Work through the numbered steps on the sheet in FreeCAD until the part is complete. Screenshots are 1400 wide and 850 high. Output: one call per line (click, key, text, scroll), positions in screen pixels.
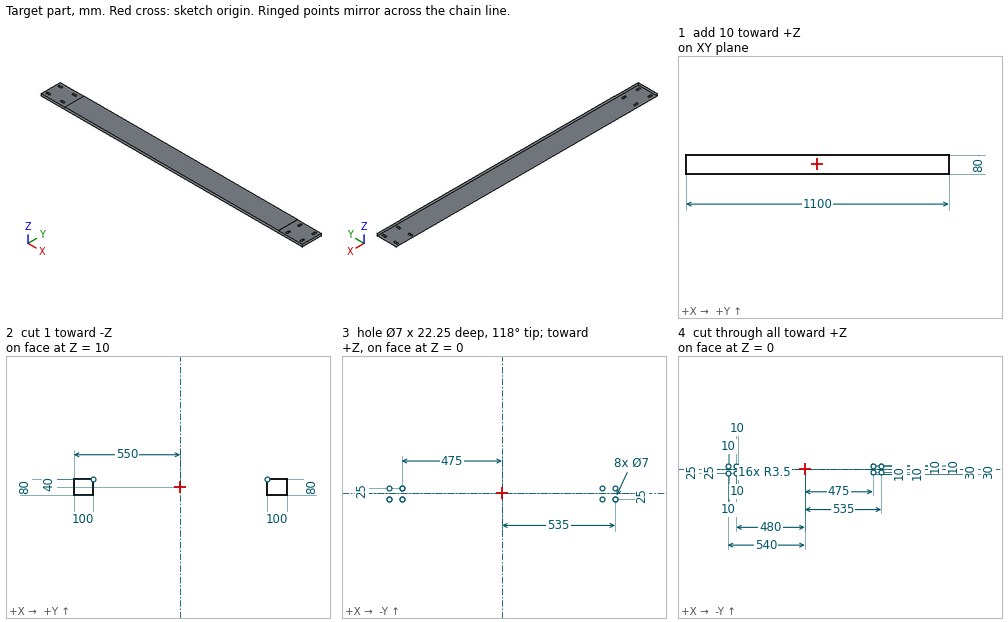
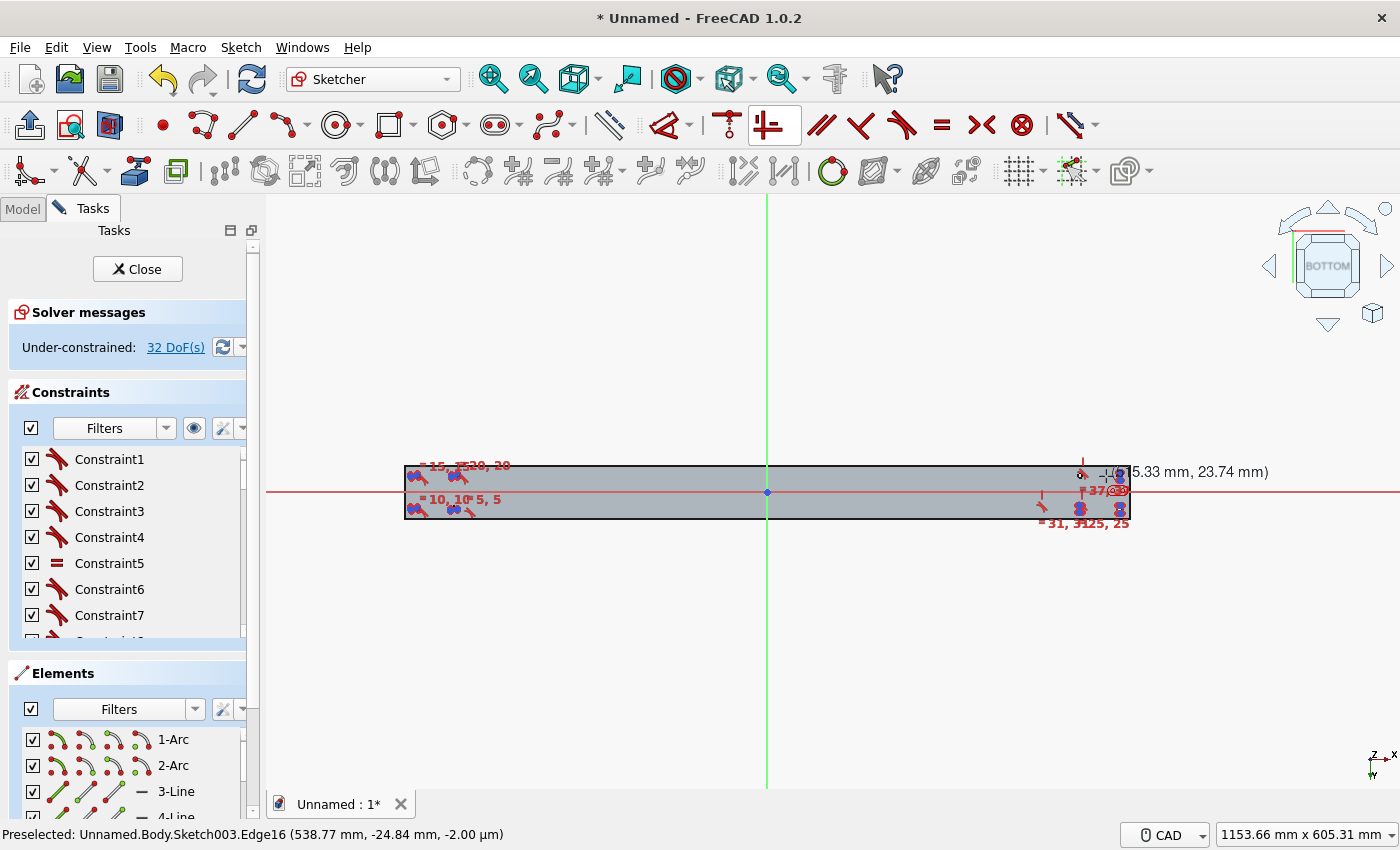
click(1080, 479)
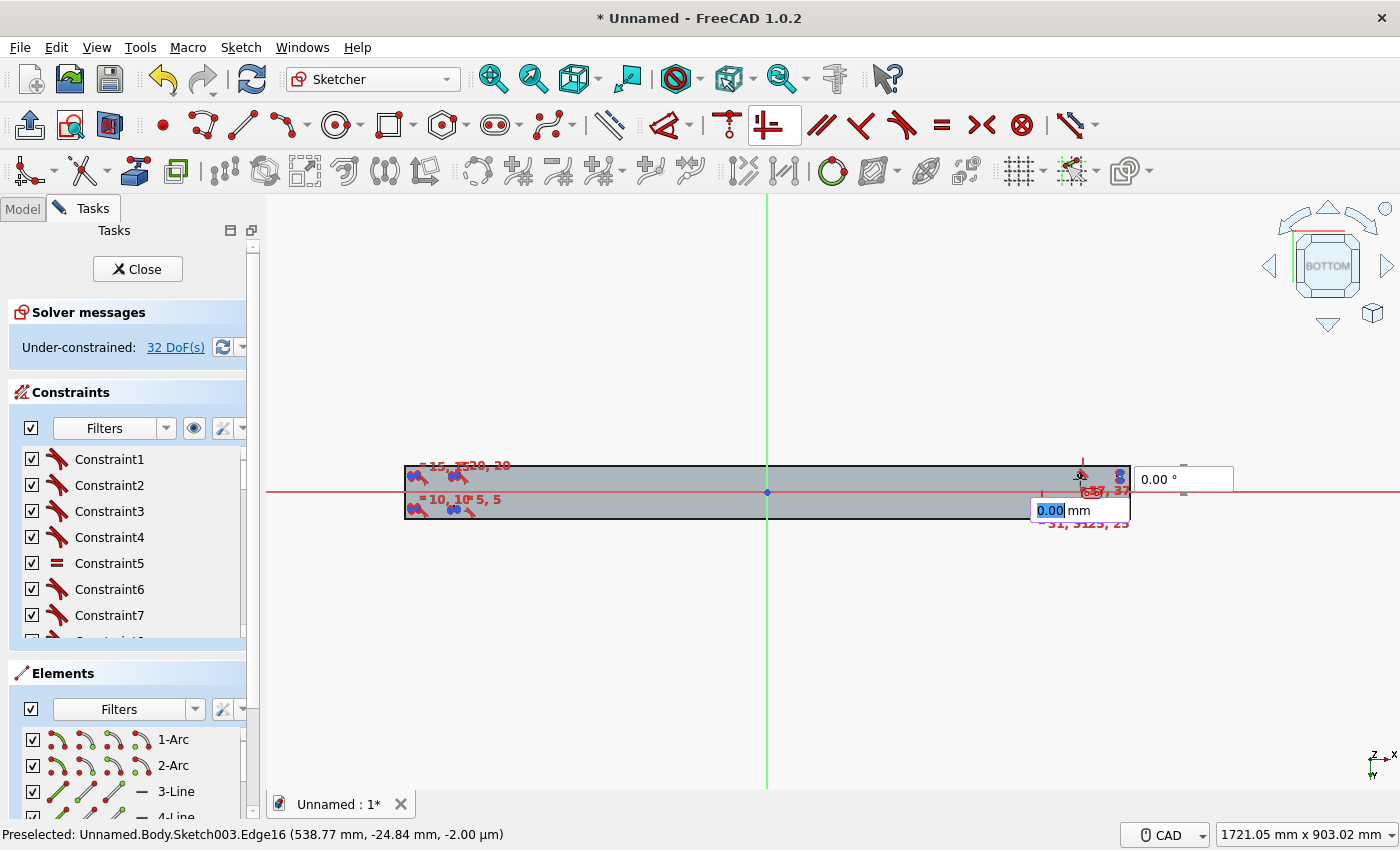
scroll(1080, 472, up, 5)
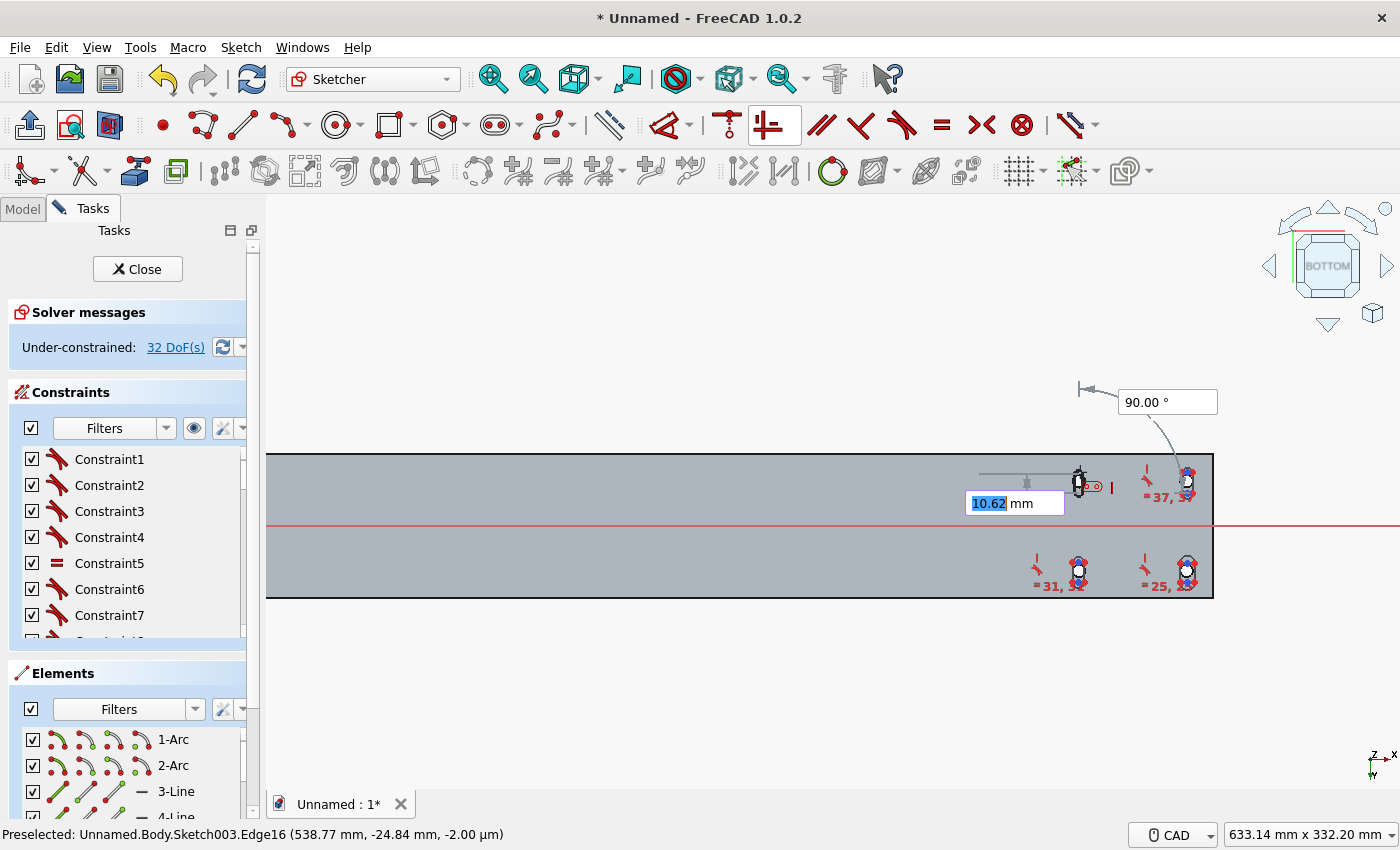
click(1079, 472)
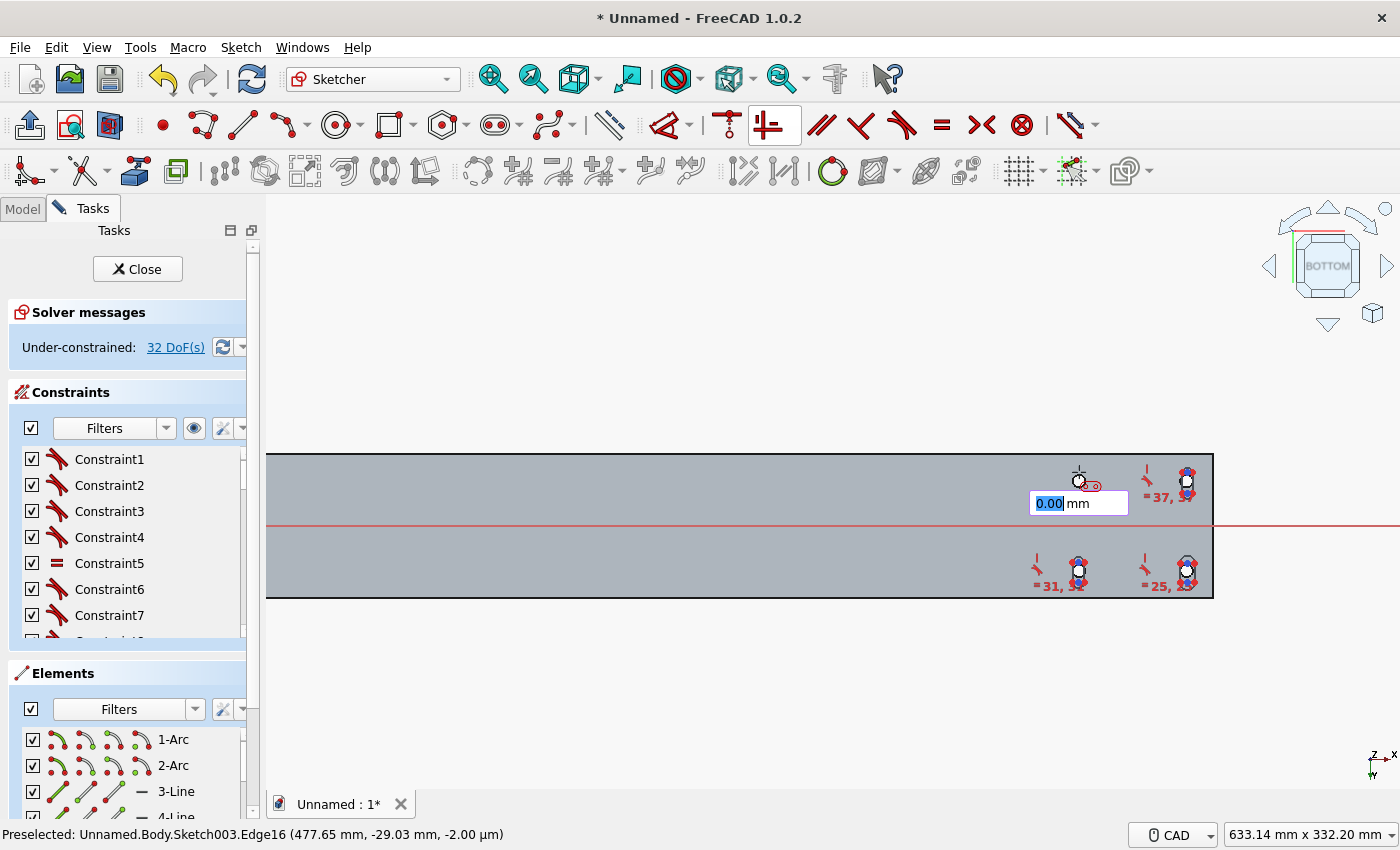
scroll(1085, 481, up, 5)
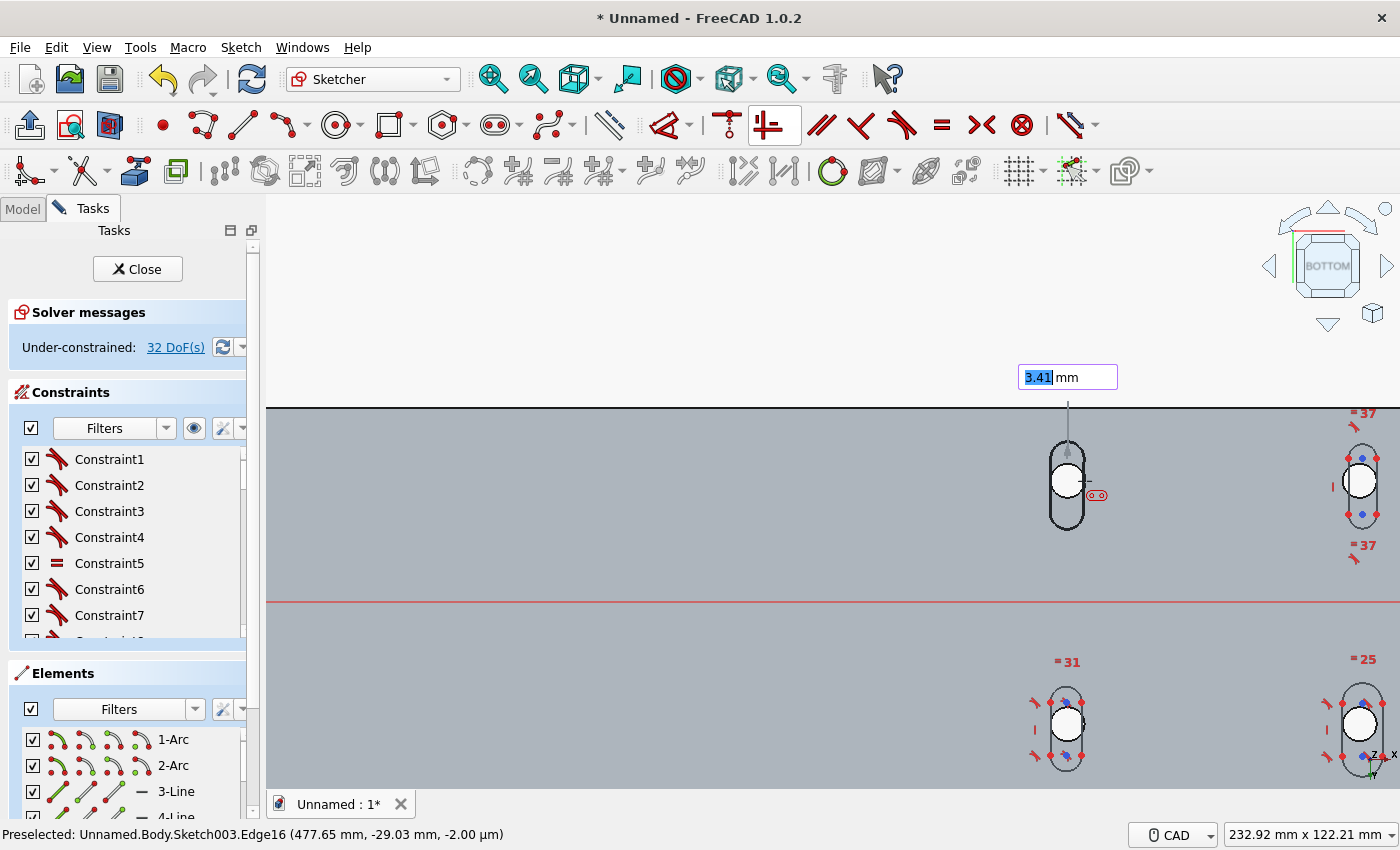
click(1085, 481)
key(Escape)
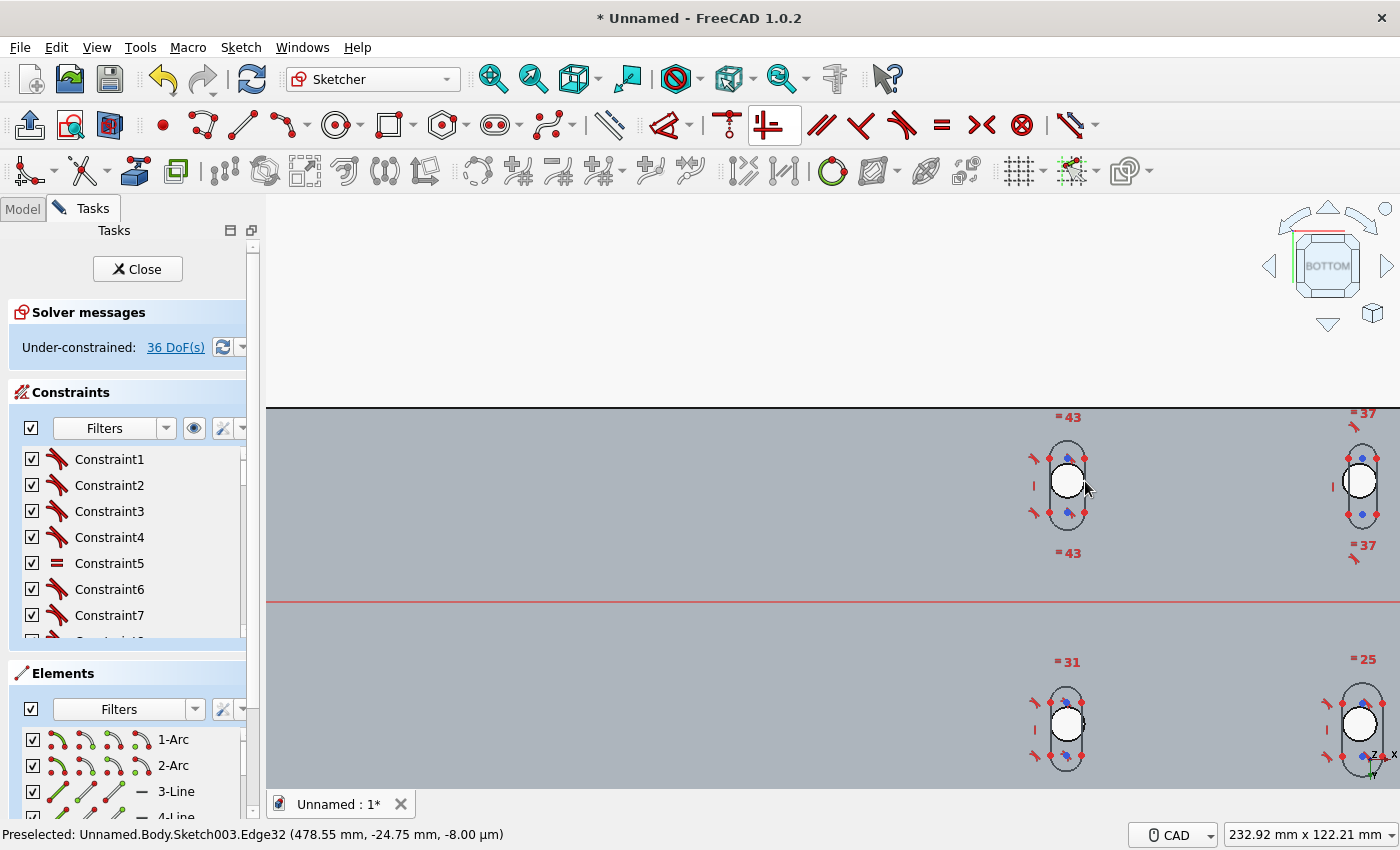
scroll(1081, 474, down, 10)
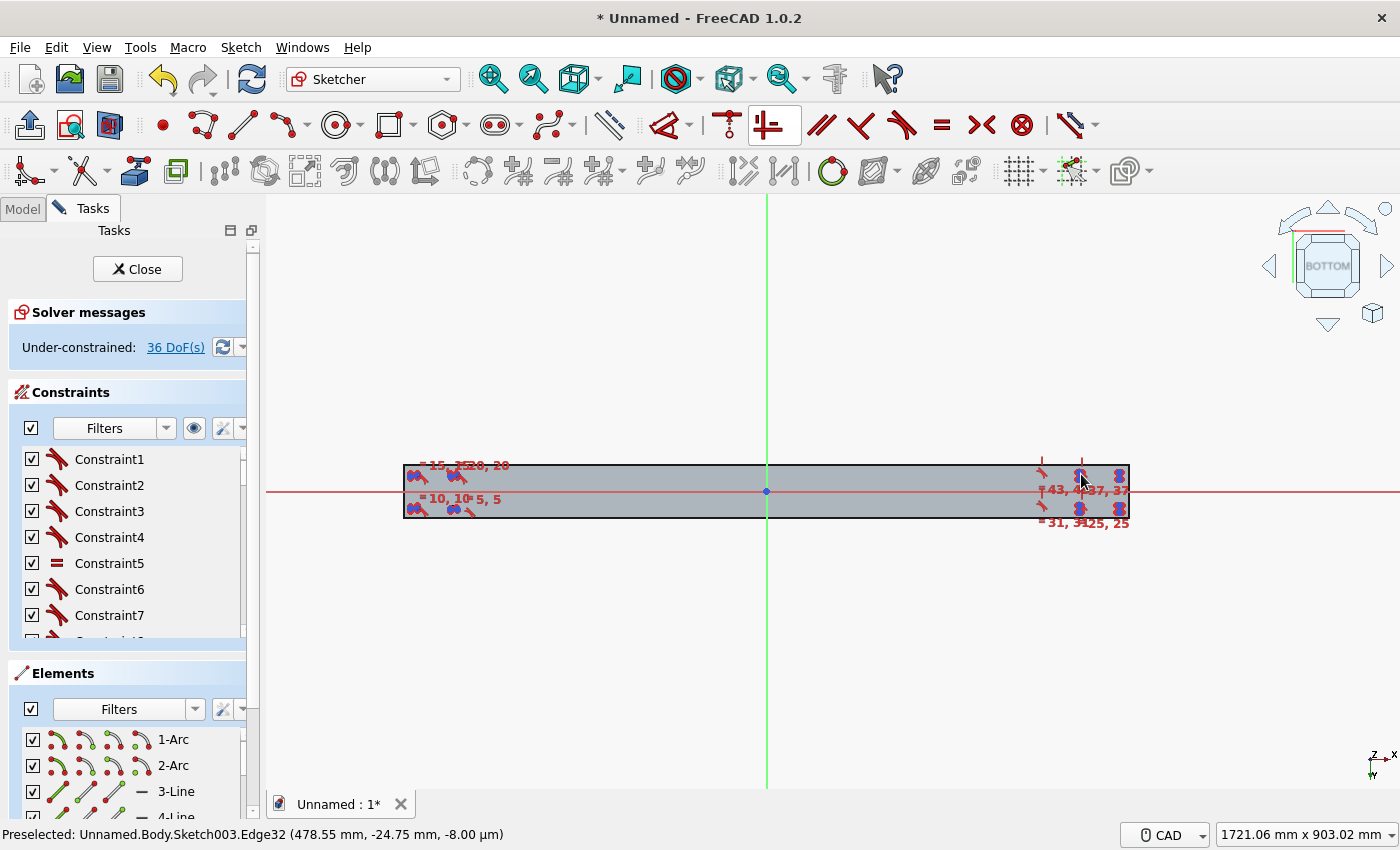
scroll(452, 508, up, 10)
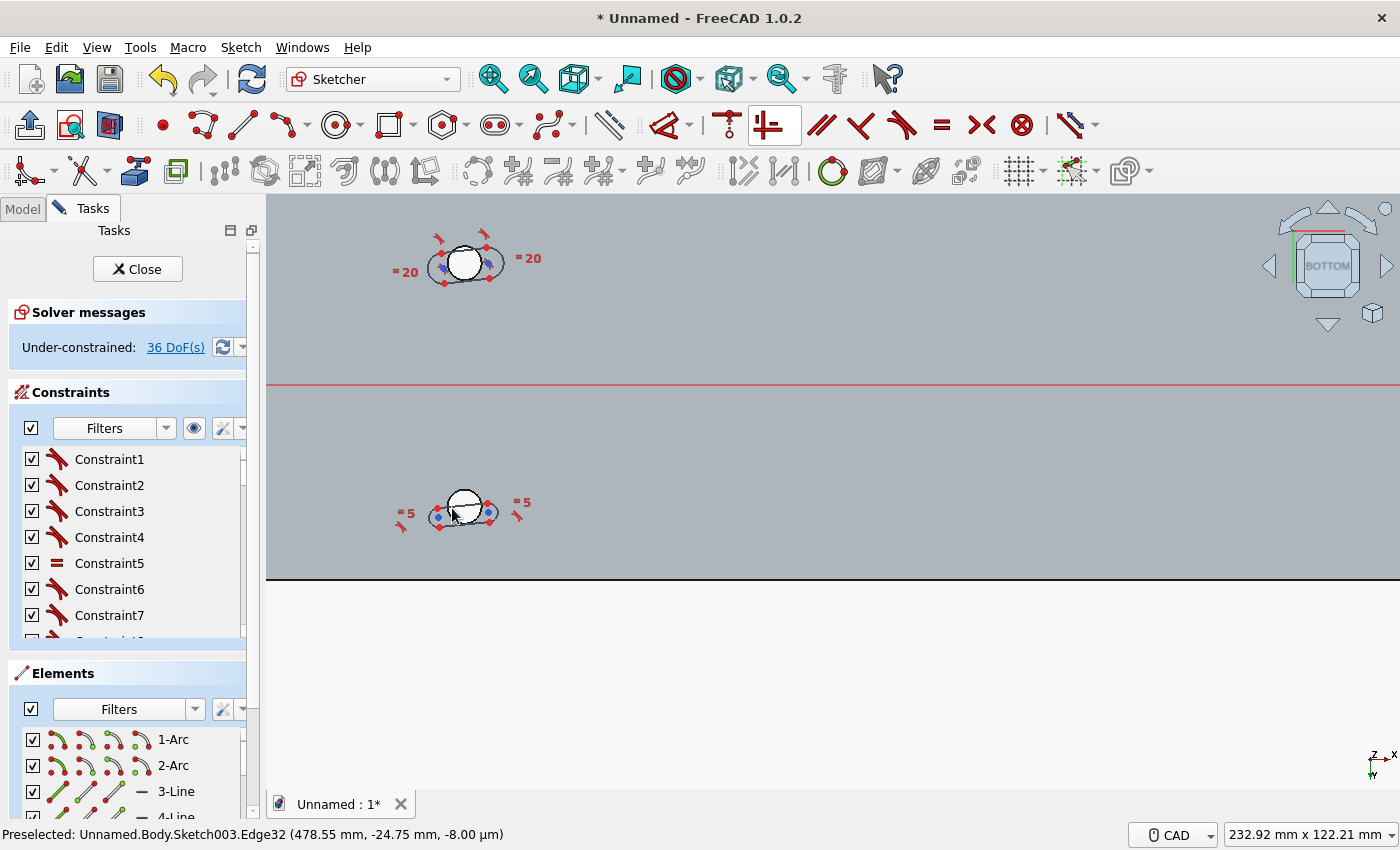
click(453, 507)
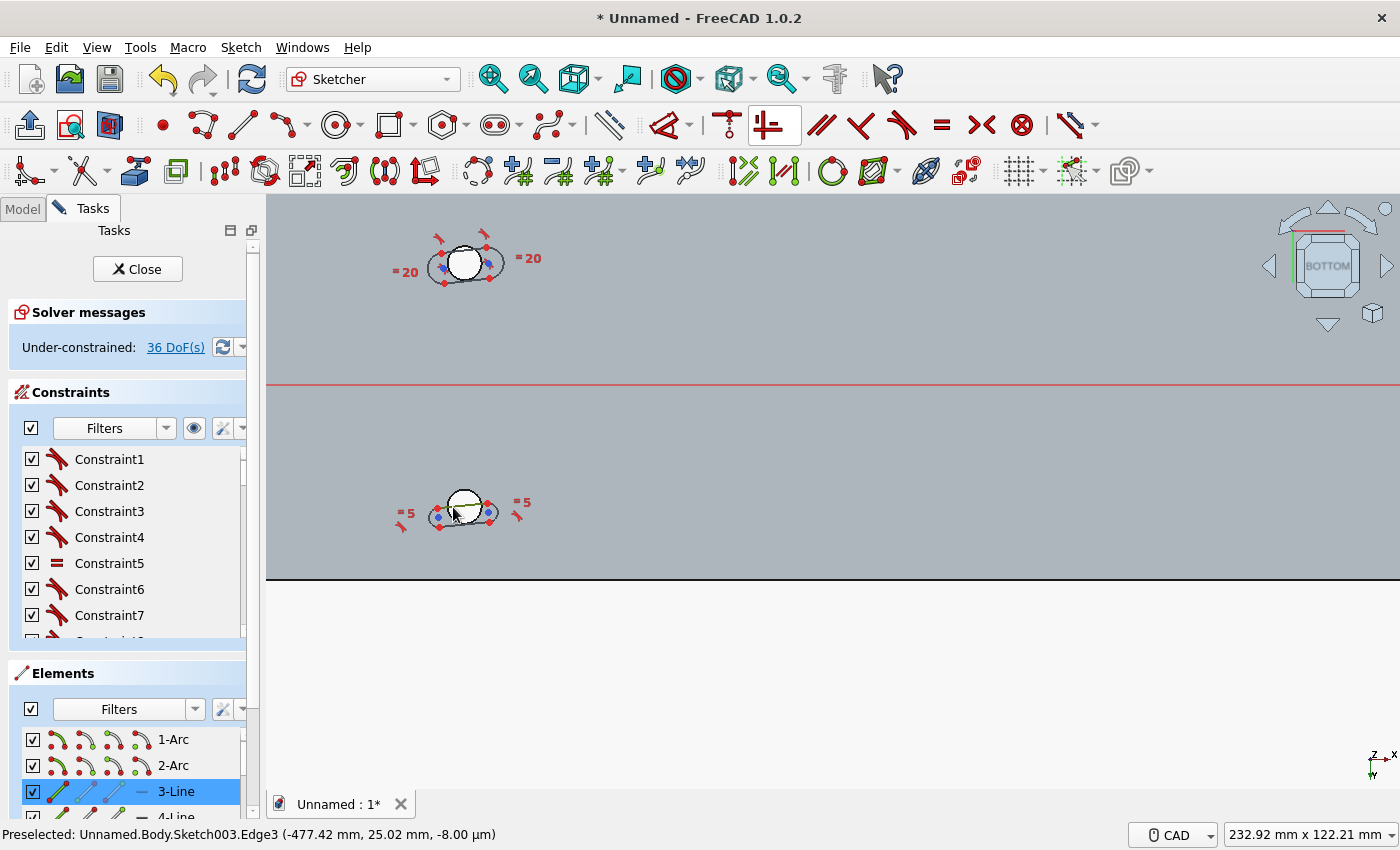
click(796, 126)